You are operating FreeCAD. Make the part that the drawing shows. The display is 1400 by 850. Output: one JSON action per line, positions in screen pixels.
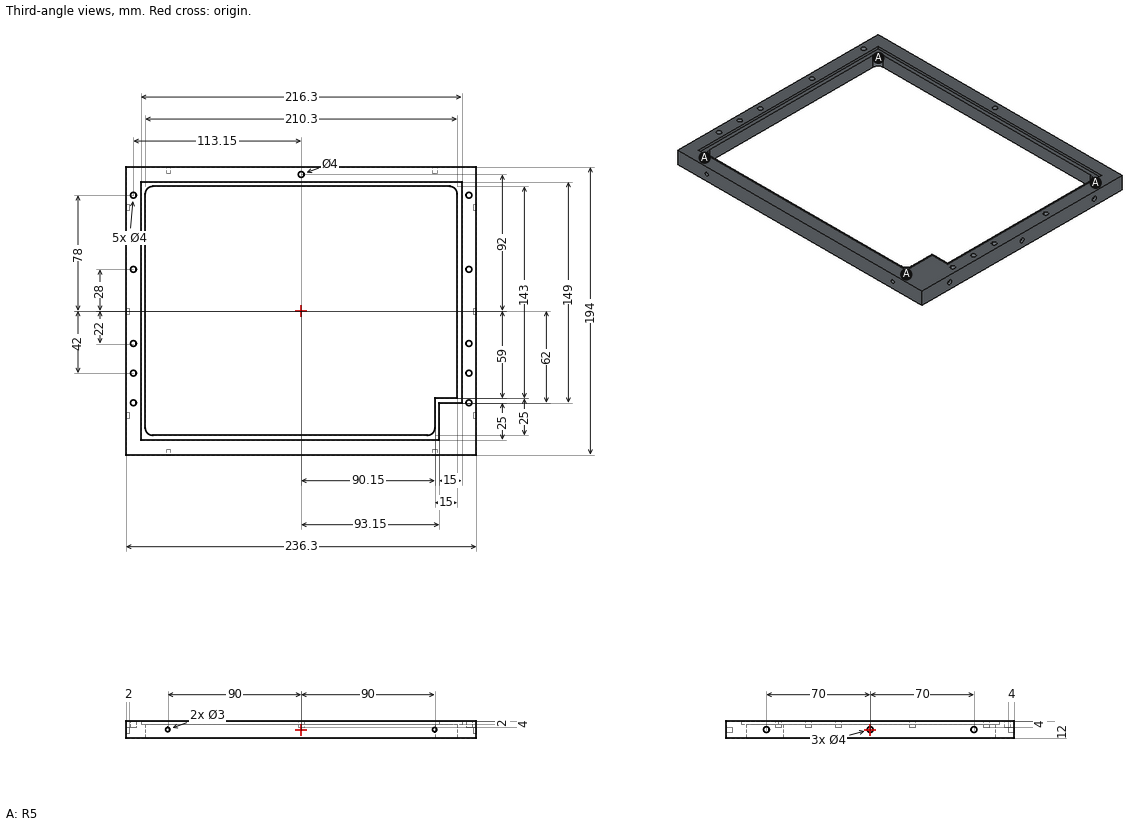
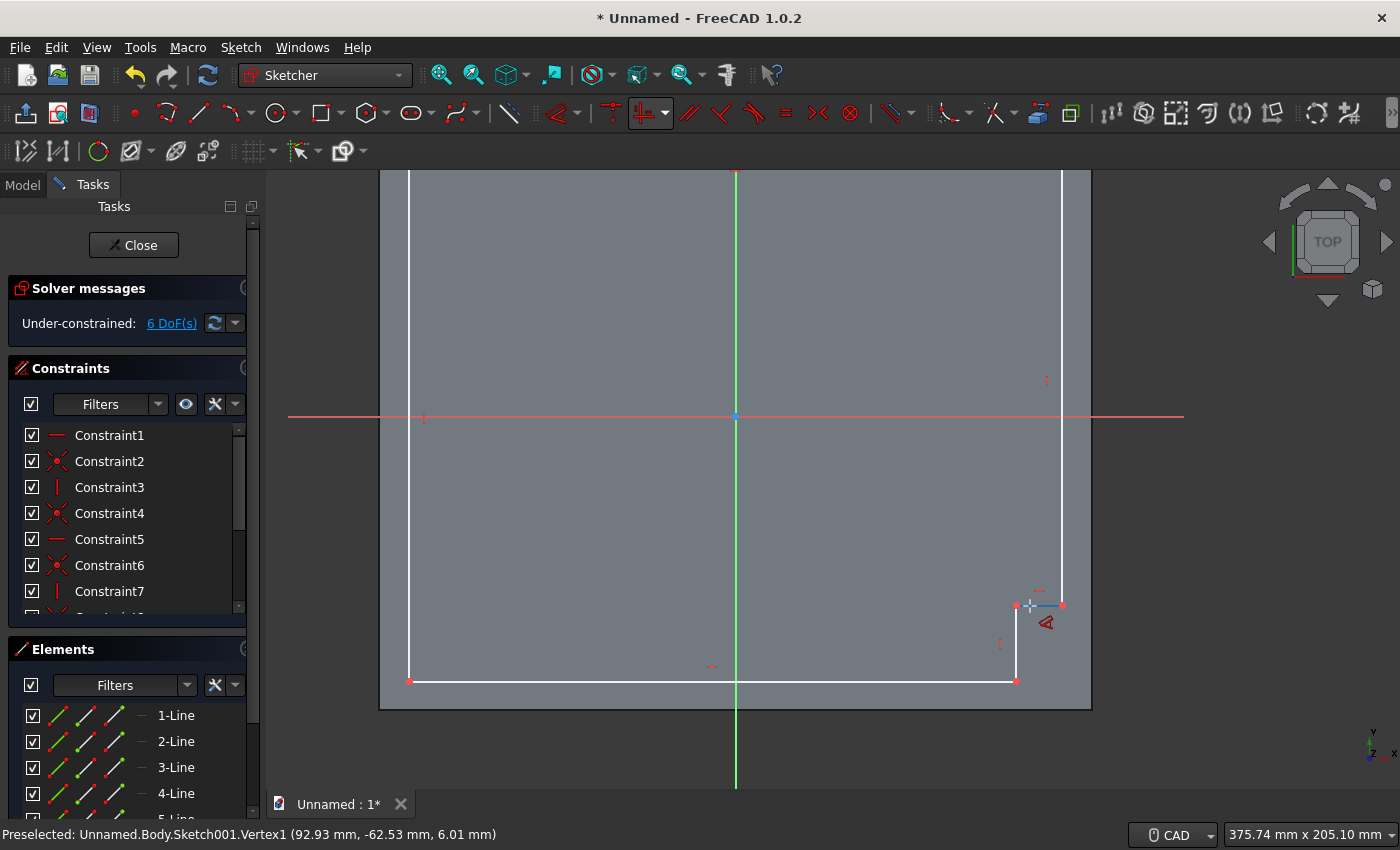
{"action": "left_click", "coordinate": [1030, 606]}
{"action": "left_click", "coordinate": [1039, 640]}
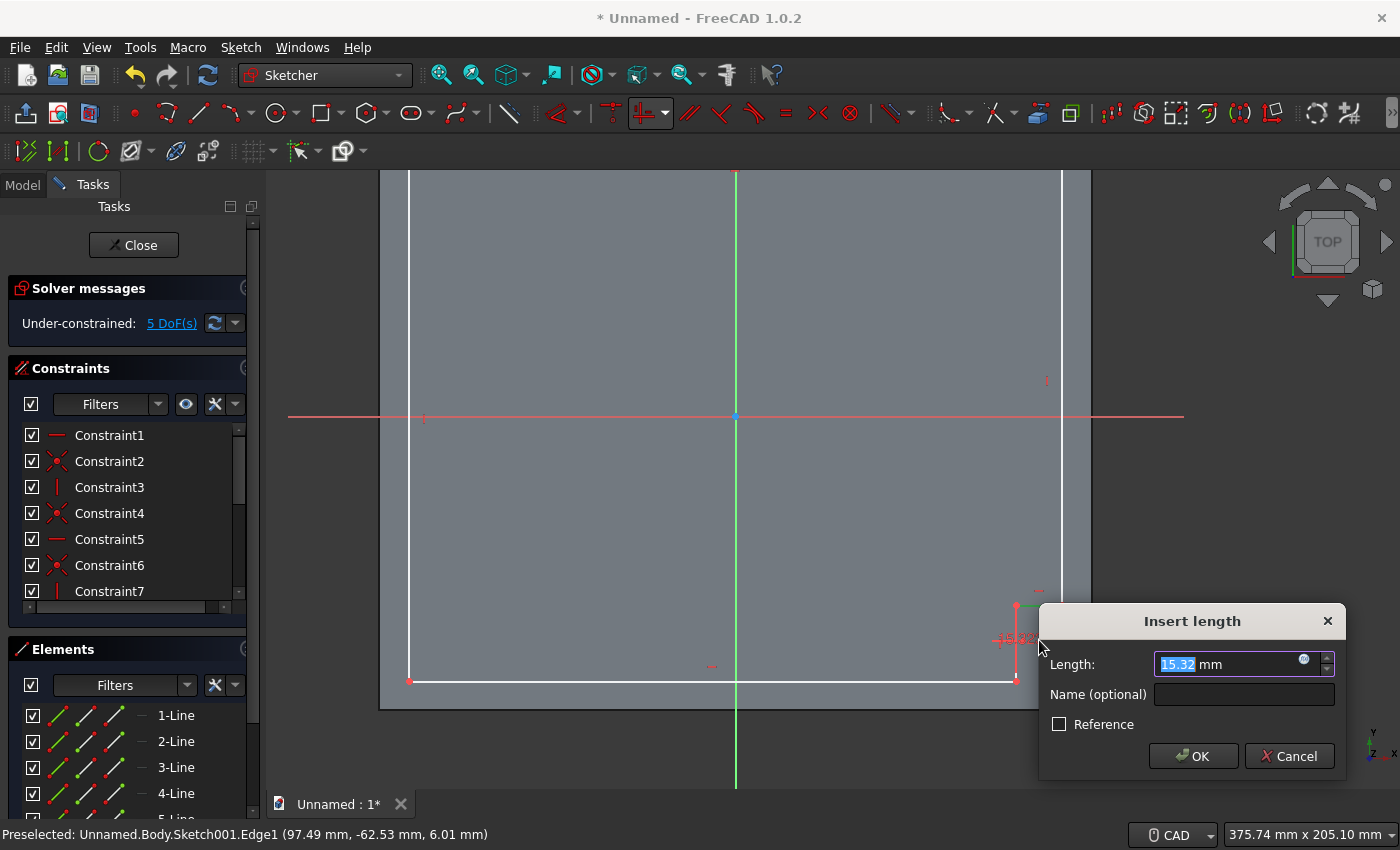
{"action": "type", "text": "15"}
{"action": "key", "text": "Return"}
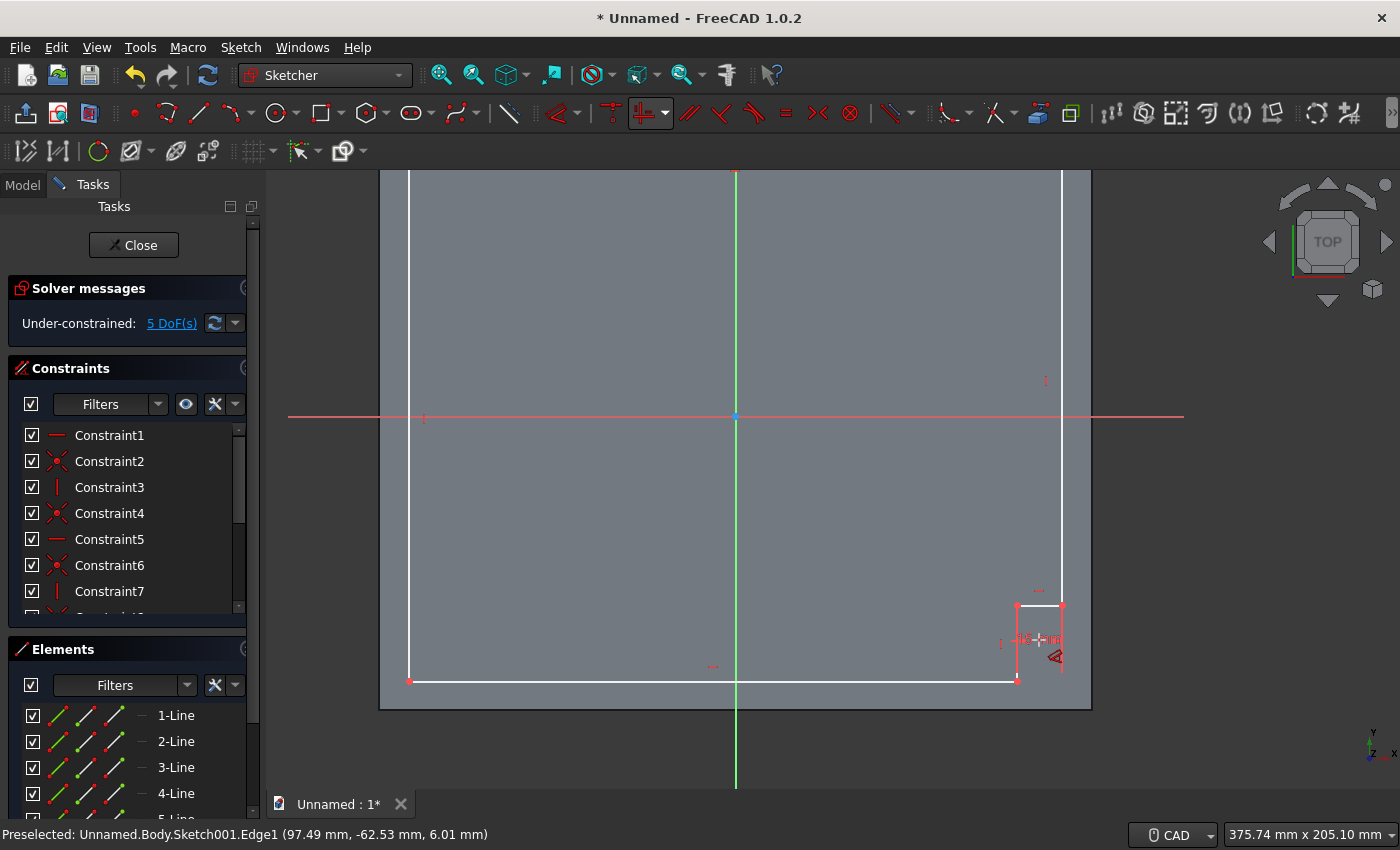
{"action": "left_click", "coordinate": [1017, 659]}
{"action": "left_click", "coordinate": [1051, 661]}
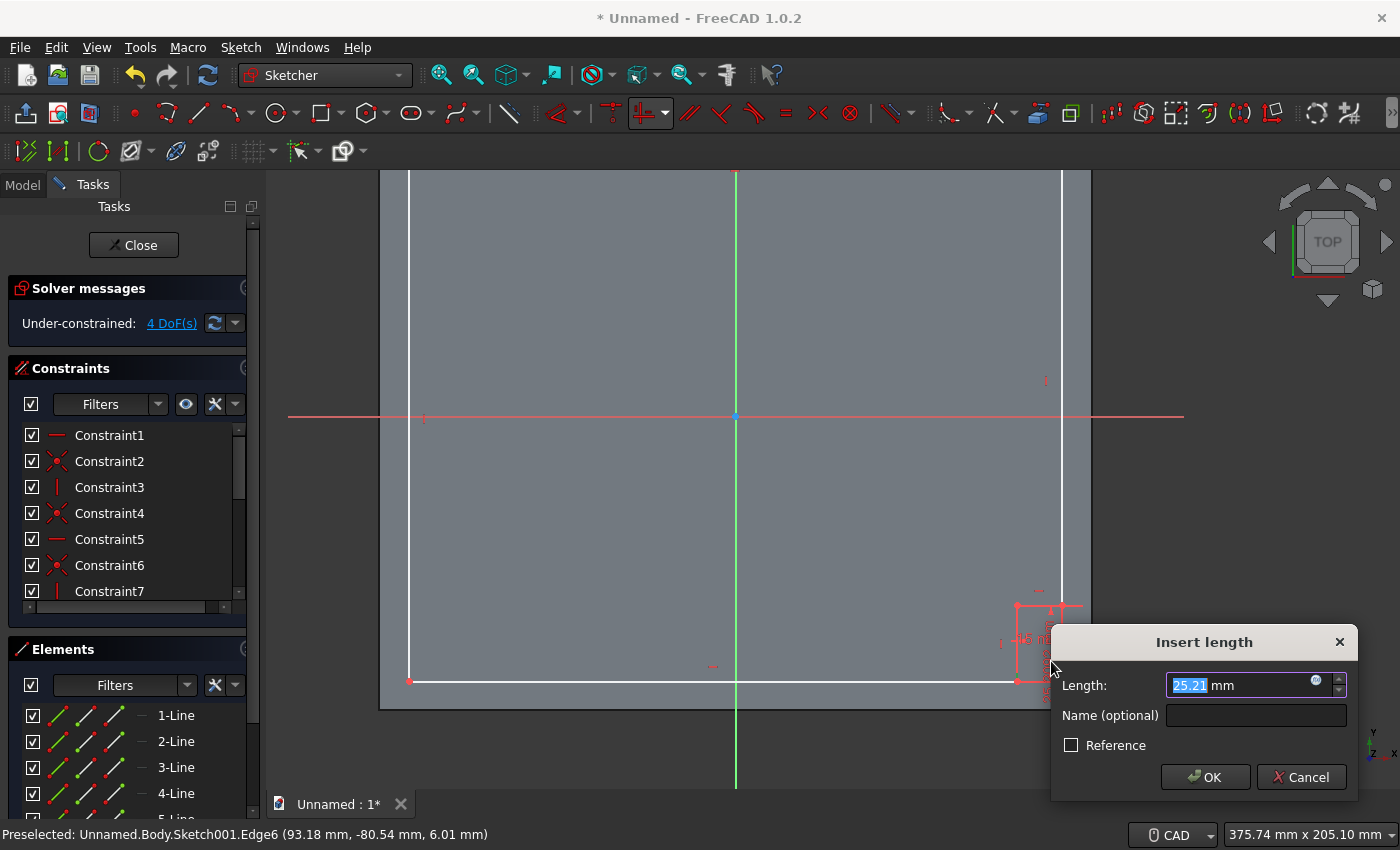
{"action": "type", "text": "25"}
{"action": "key", "text": "Return"}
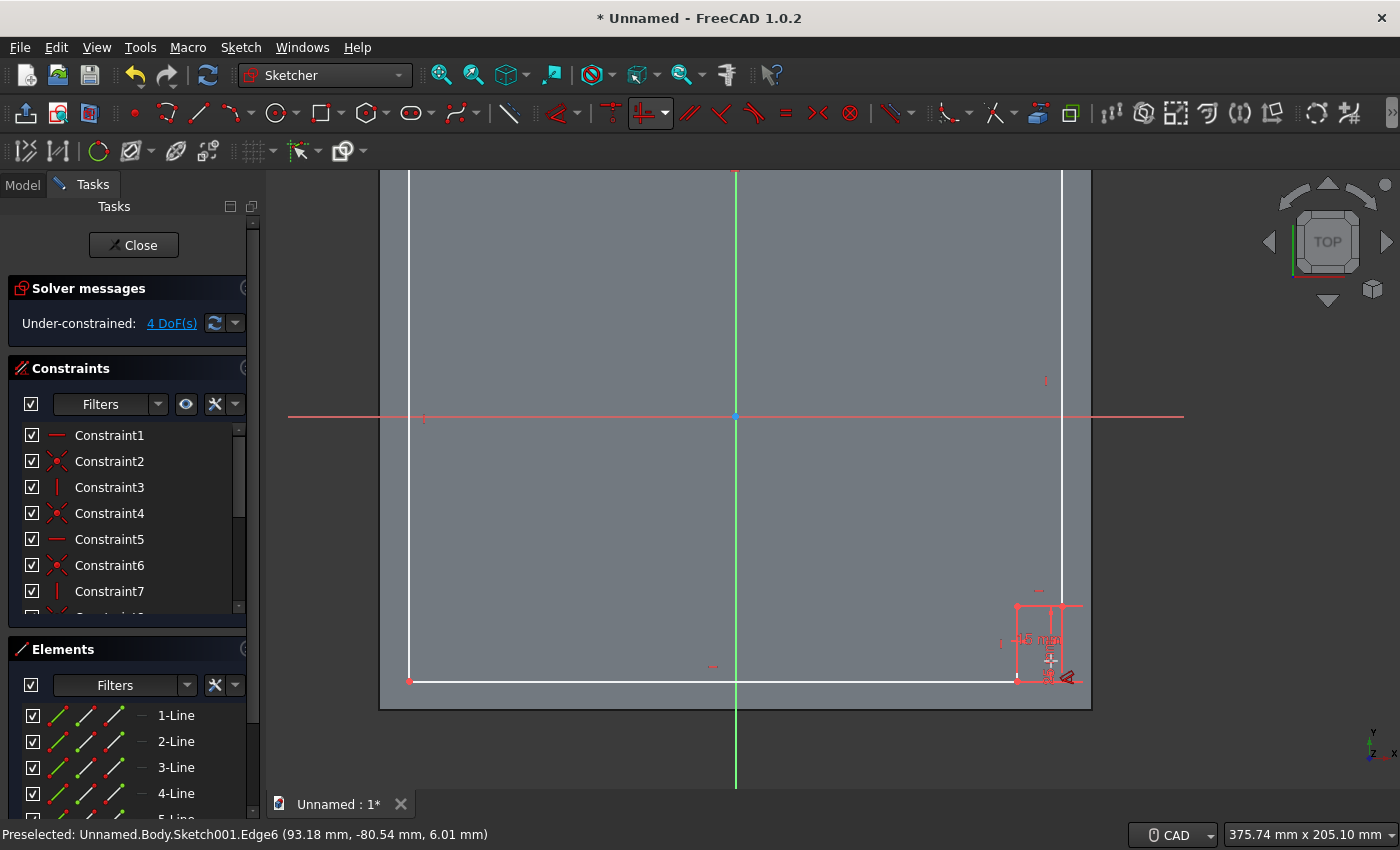
{"action": "left_click", "coordinate": [1062, 471]}
{"action": "left_click", "coordinate": [1096, 402]}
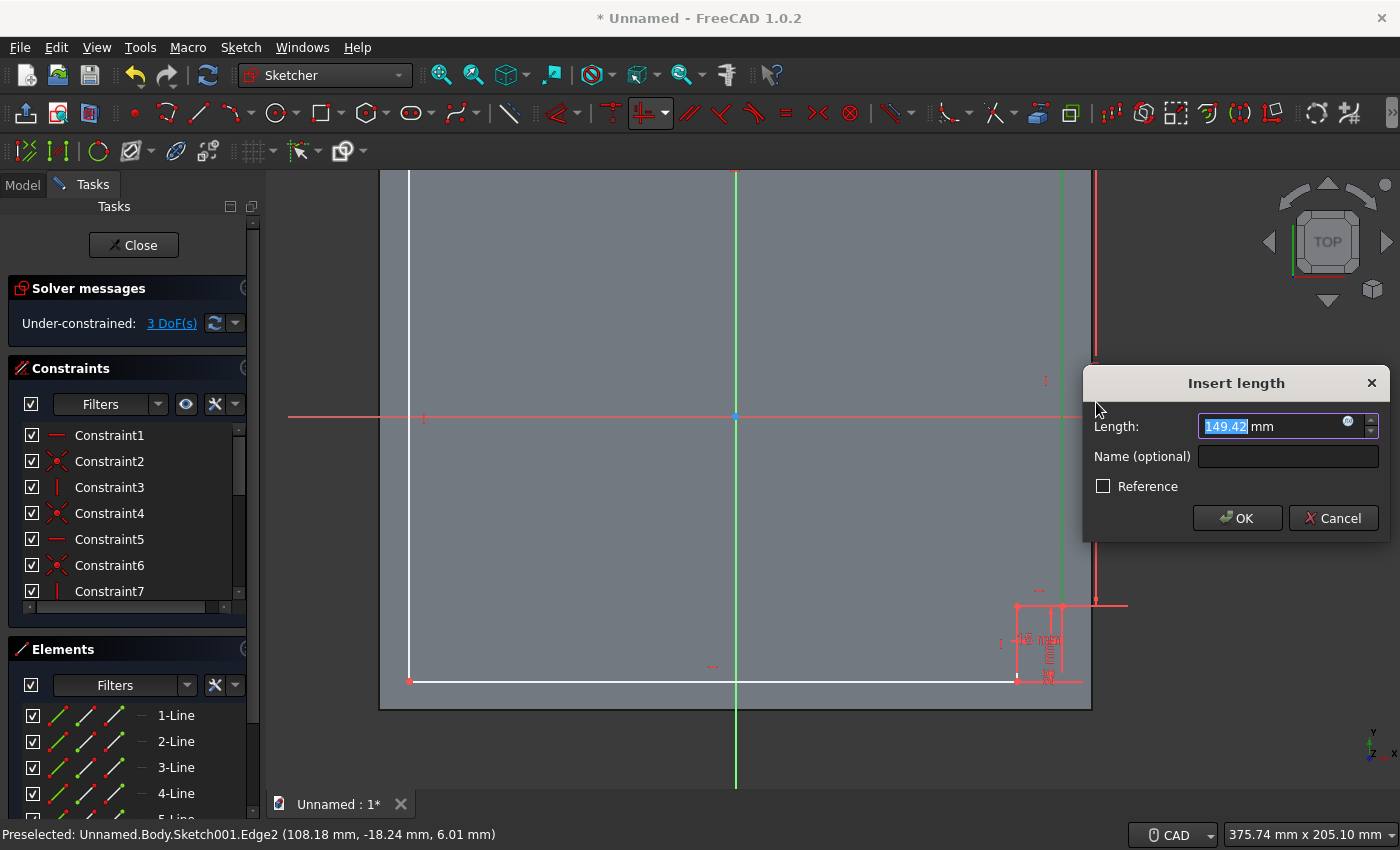
{"action": "type", "text": "149"}
{"action": "key", "text": "Return"}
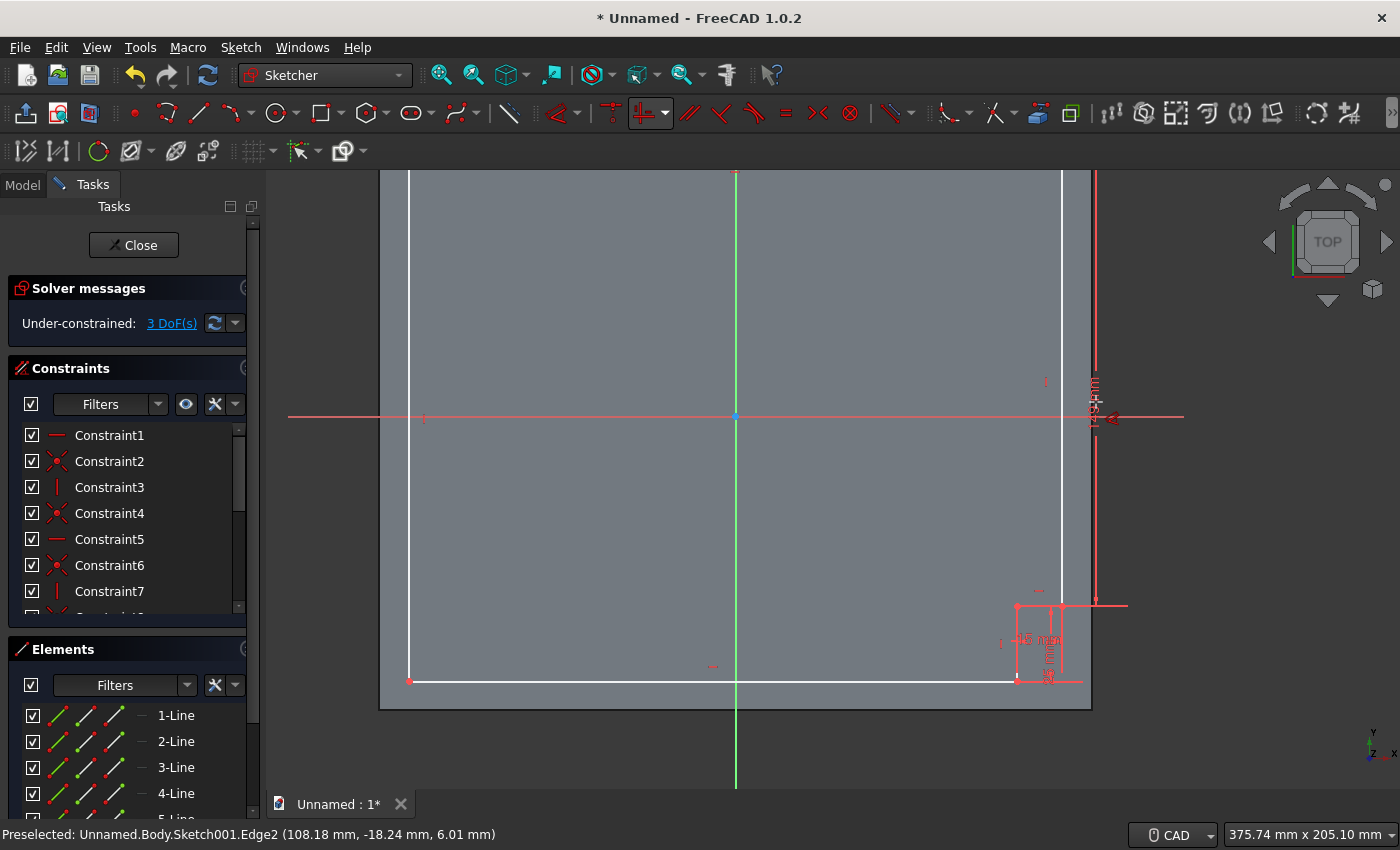
{"action": "left_click", "coordinate": [1017, 606]}
{"action": "left_click", "coordinate": [702, 511]}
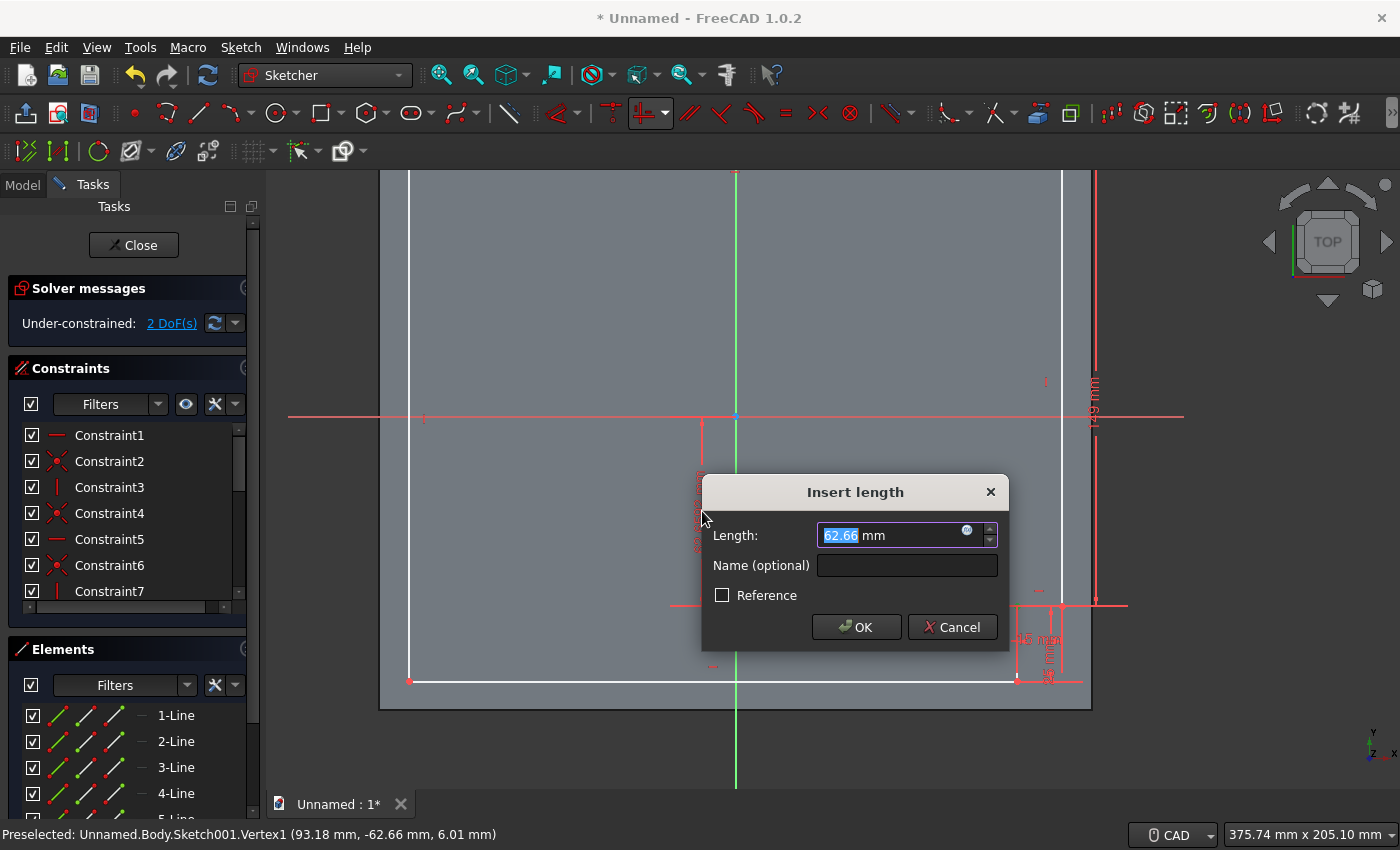
{"action": "type", "text": "62"}
{"action": "key", "text": "Return"}